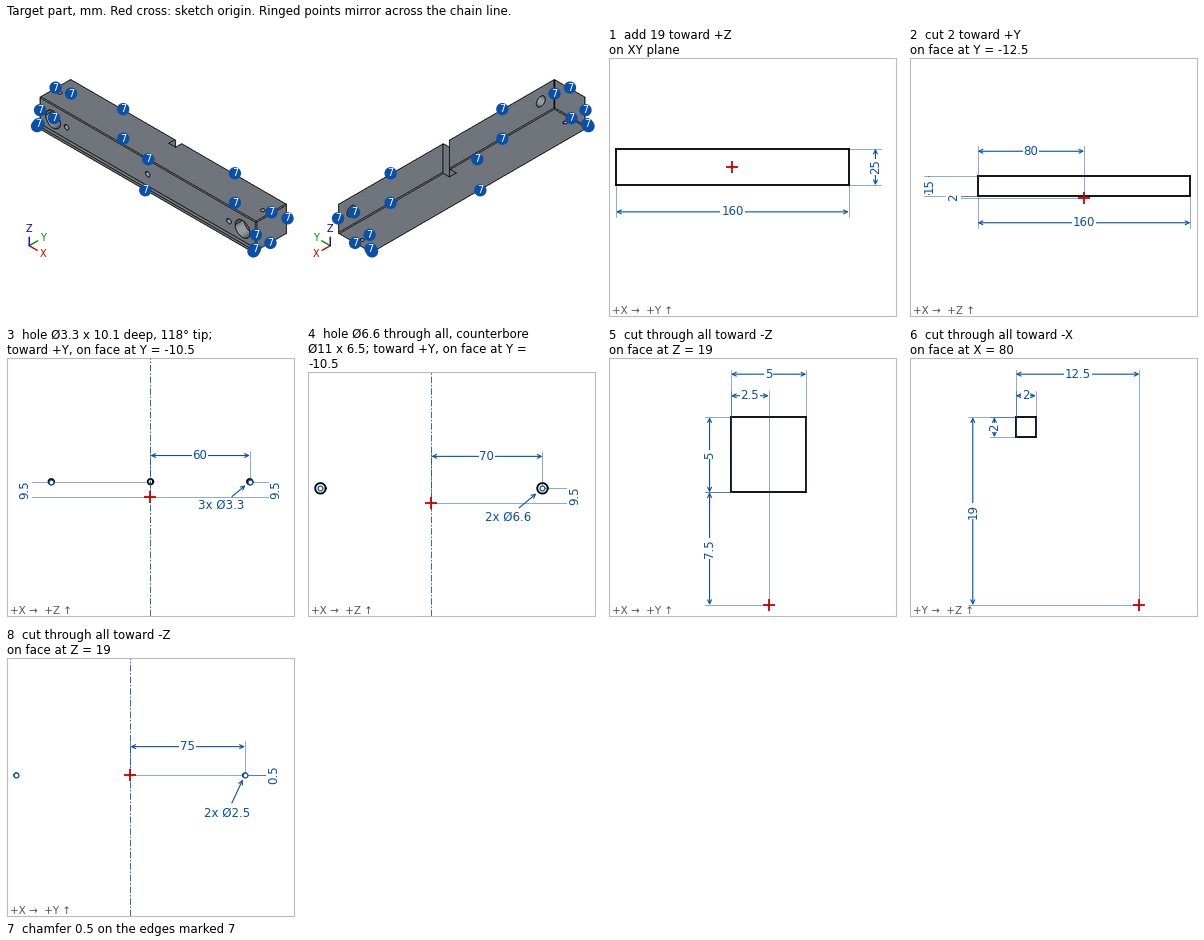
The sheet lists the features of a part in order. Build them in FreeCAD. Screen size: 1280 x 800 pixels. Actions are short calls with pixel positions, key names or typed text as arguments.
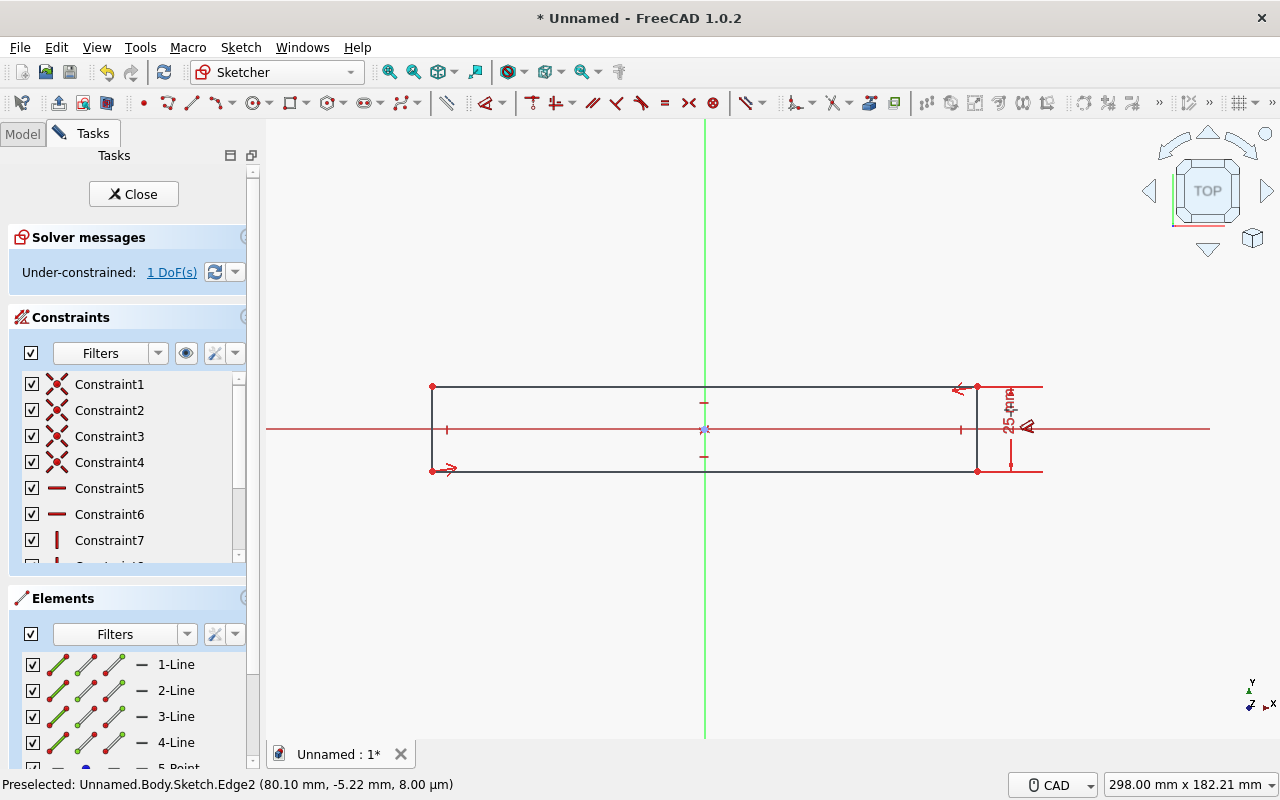
click(596, 472)
click(579, 506)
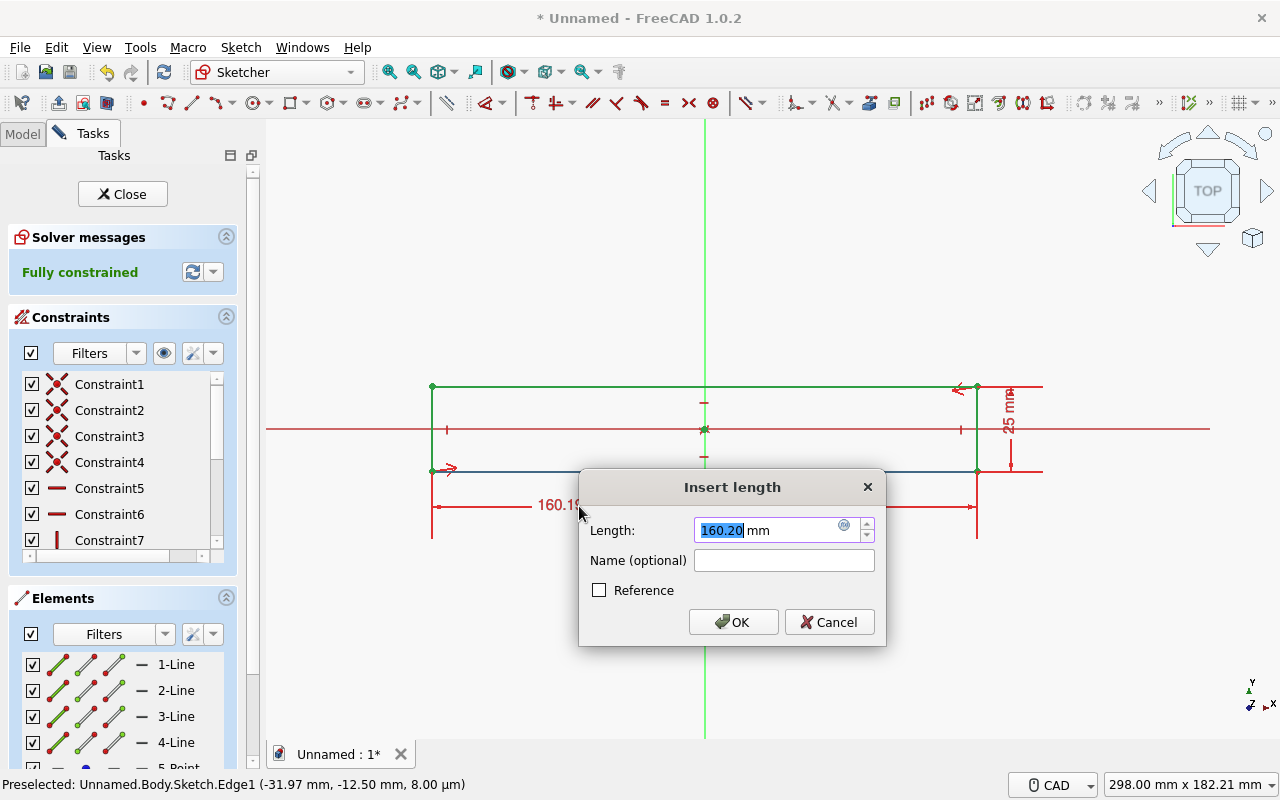
text(160)
key(Return)
key(Escape)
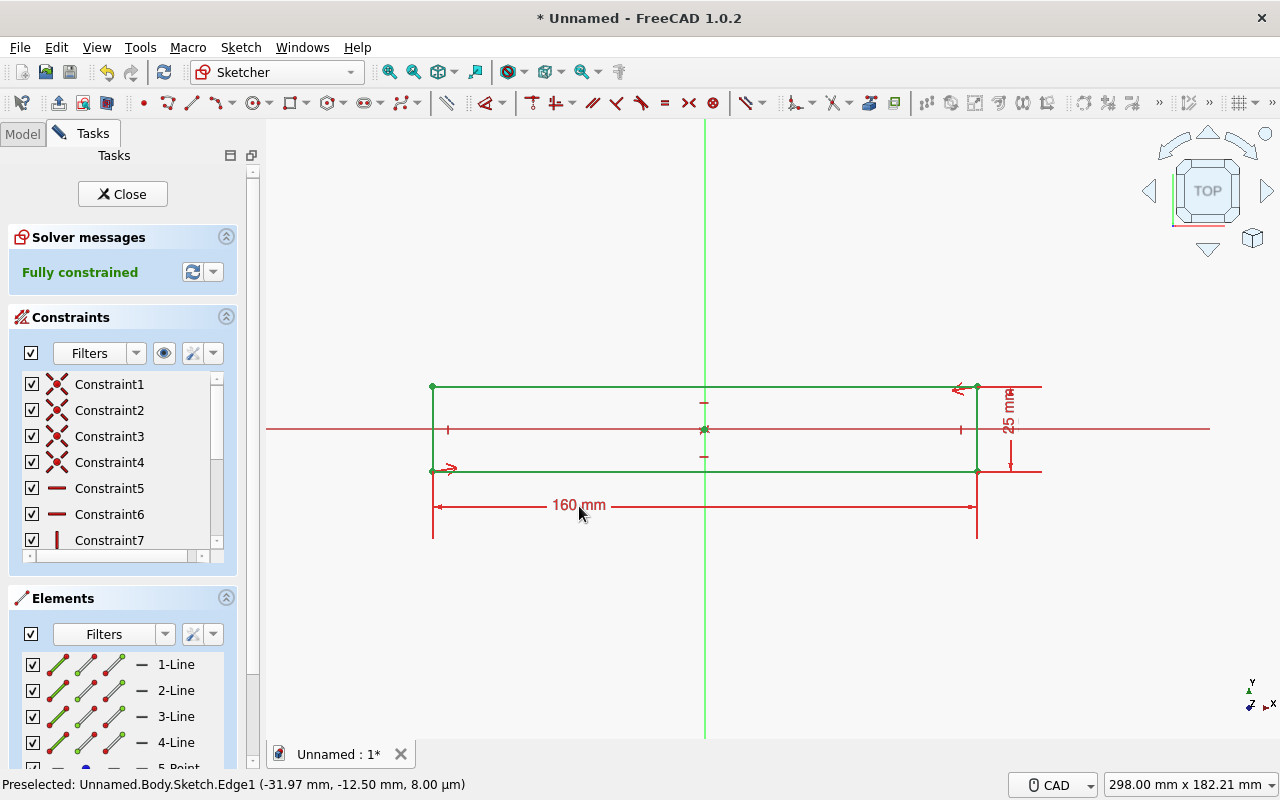
click(123, 194)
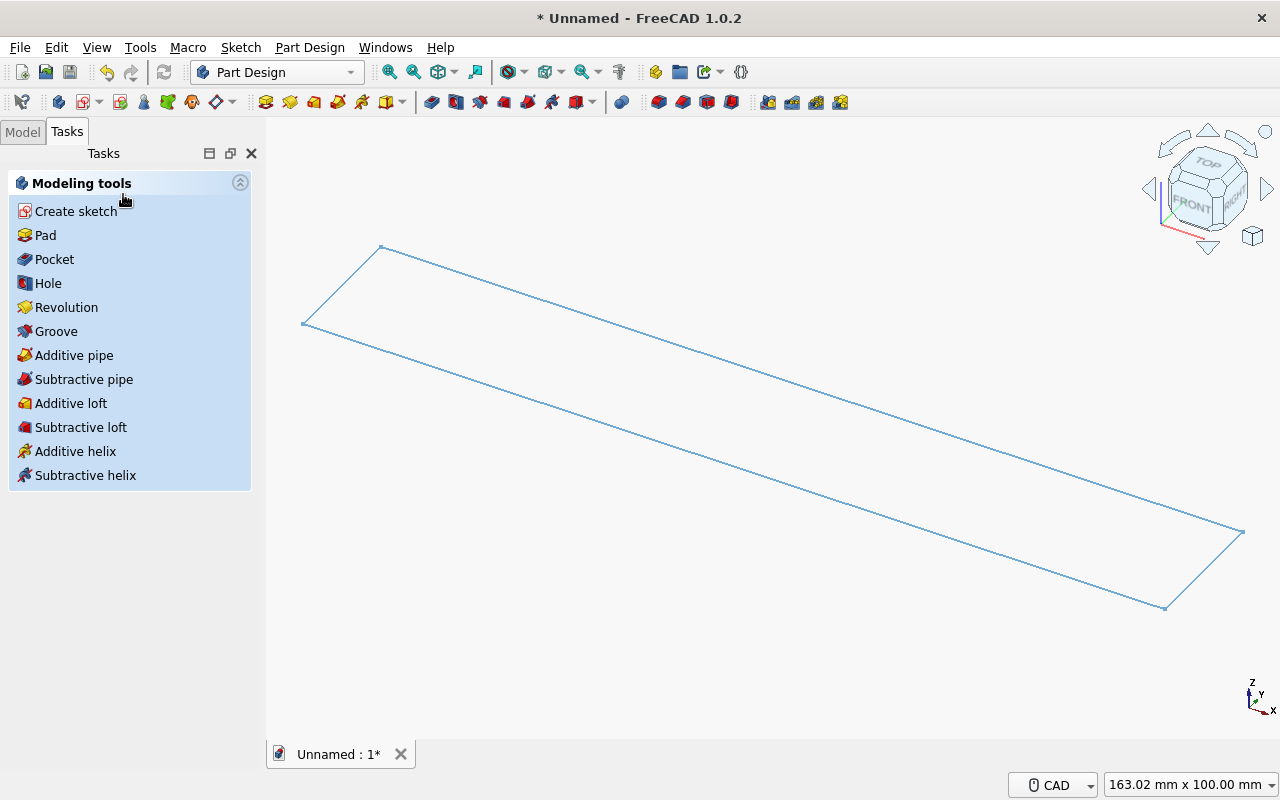
click(266, 102)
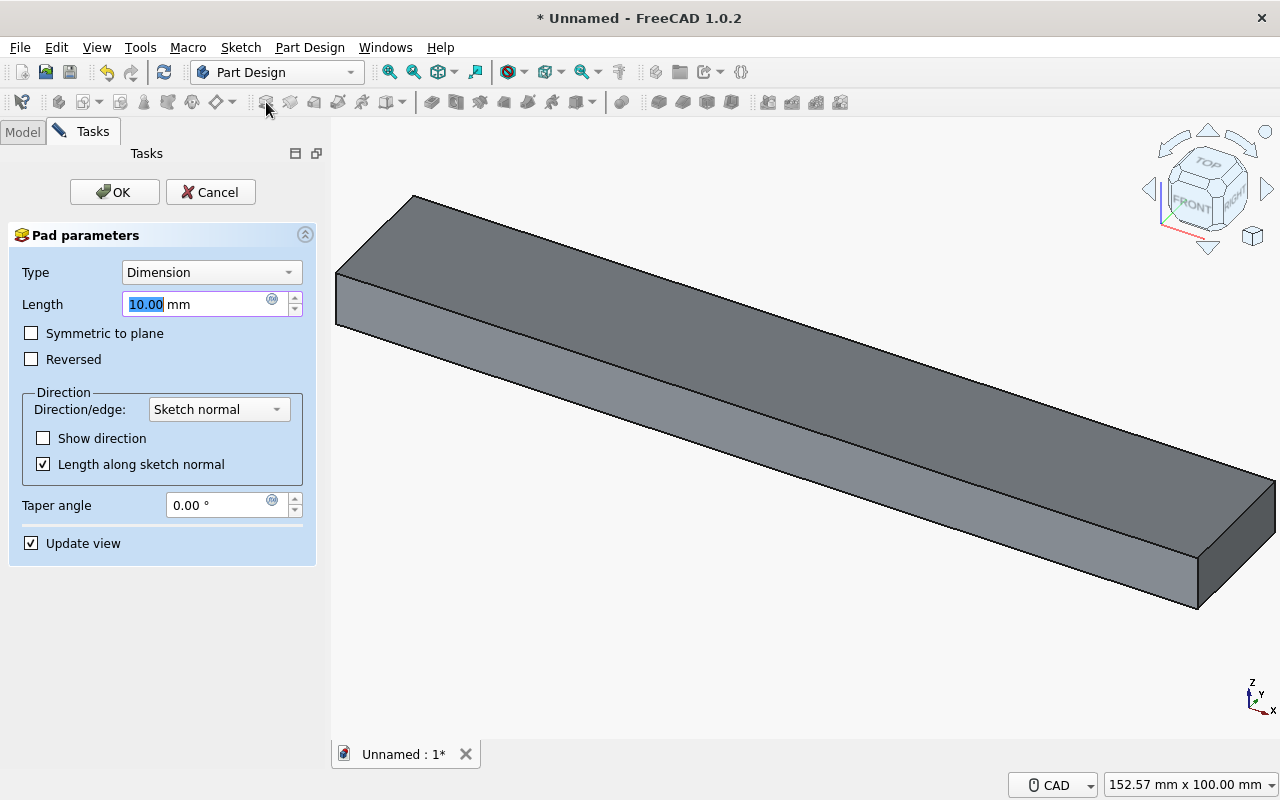
text(19)
key(Tab)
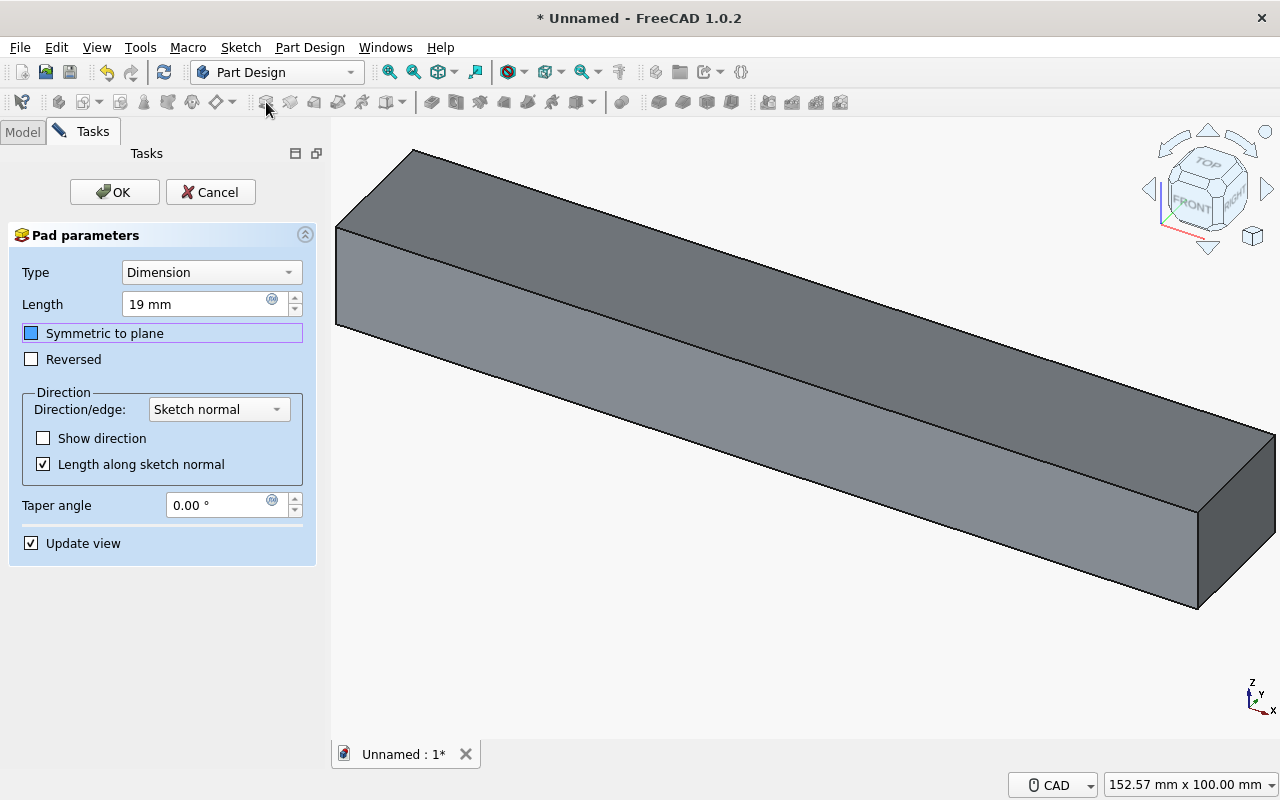
click(115, 192)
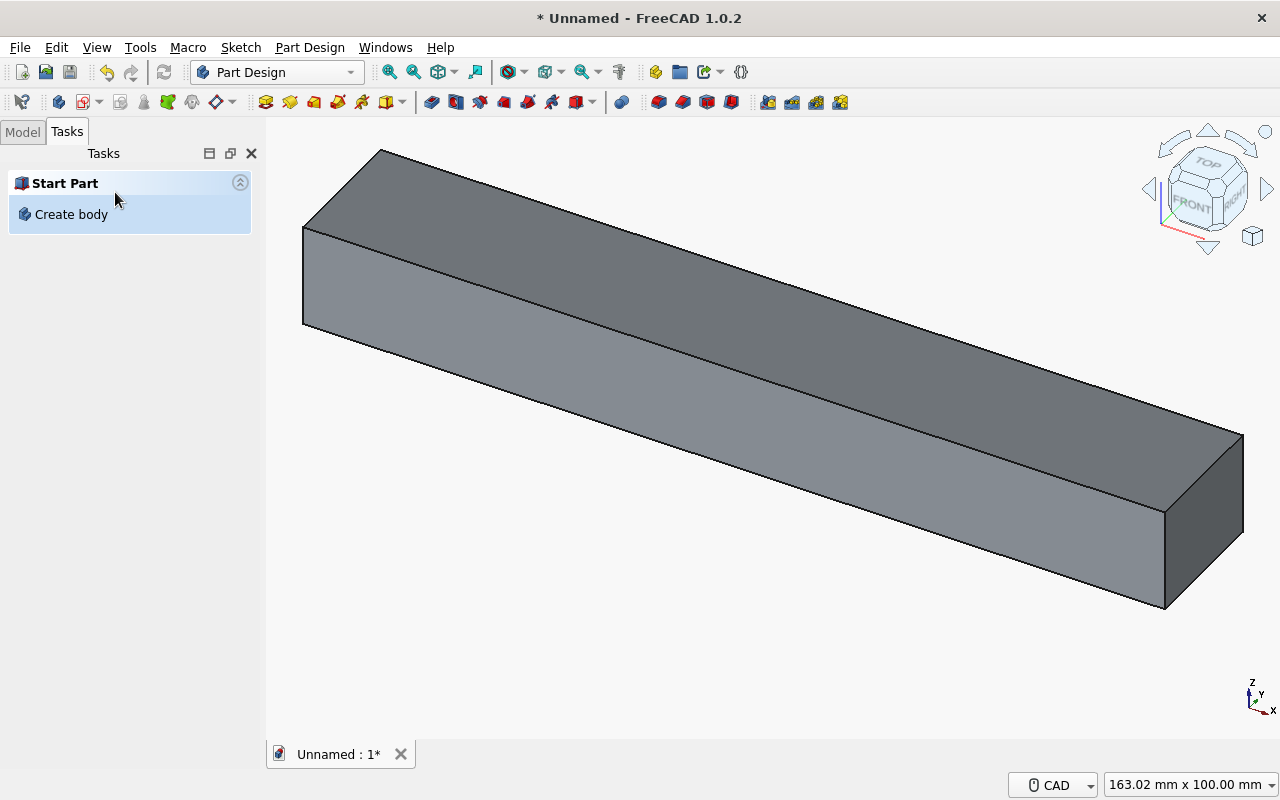
click(1103, 540)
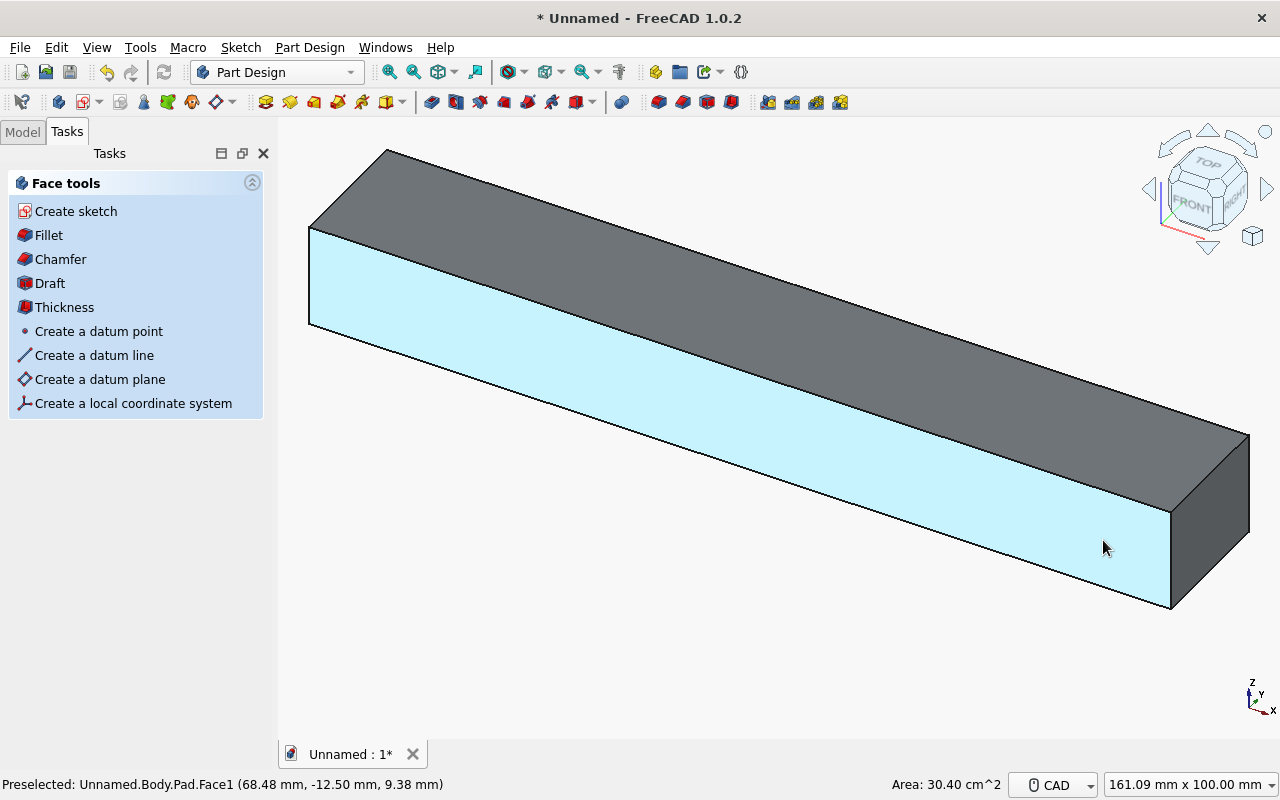
click(84, 102)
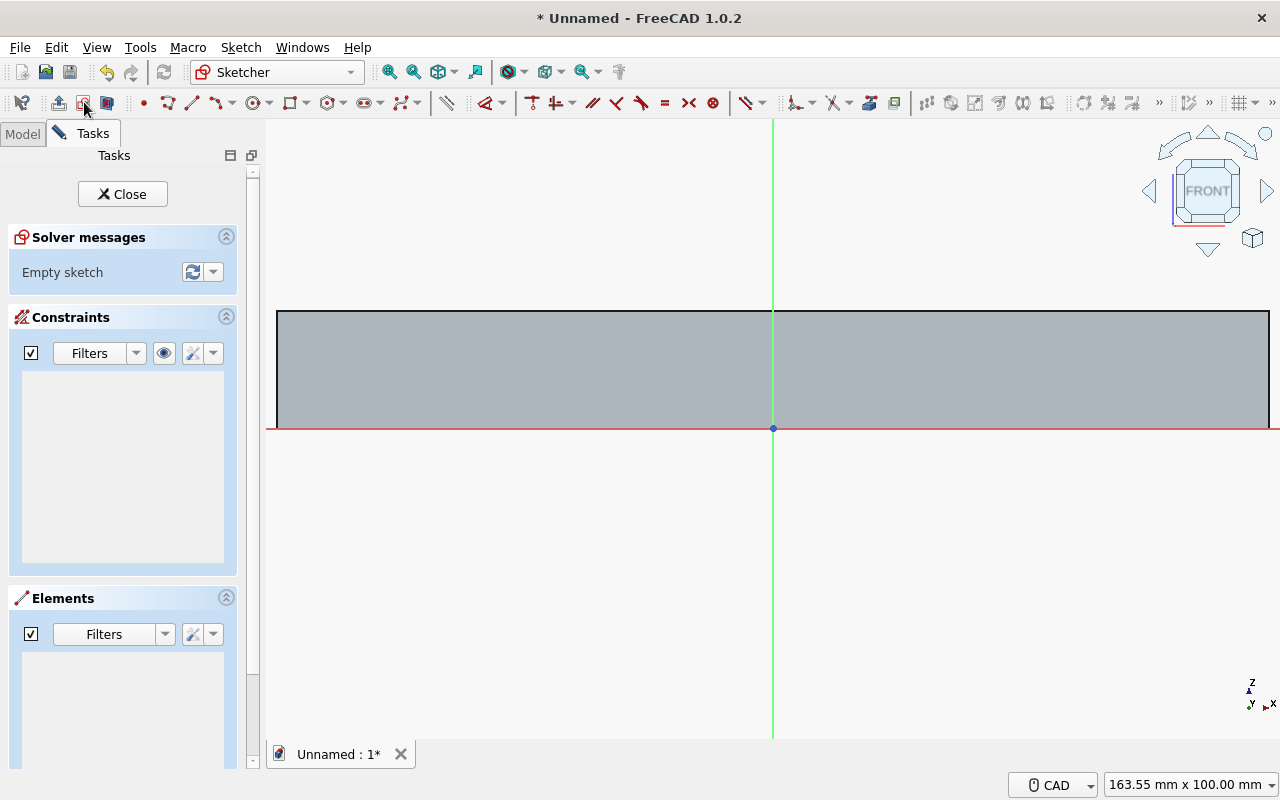
scroll(621, 493, down, 3)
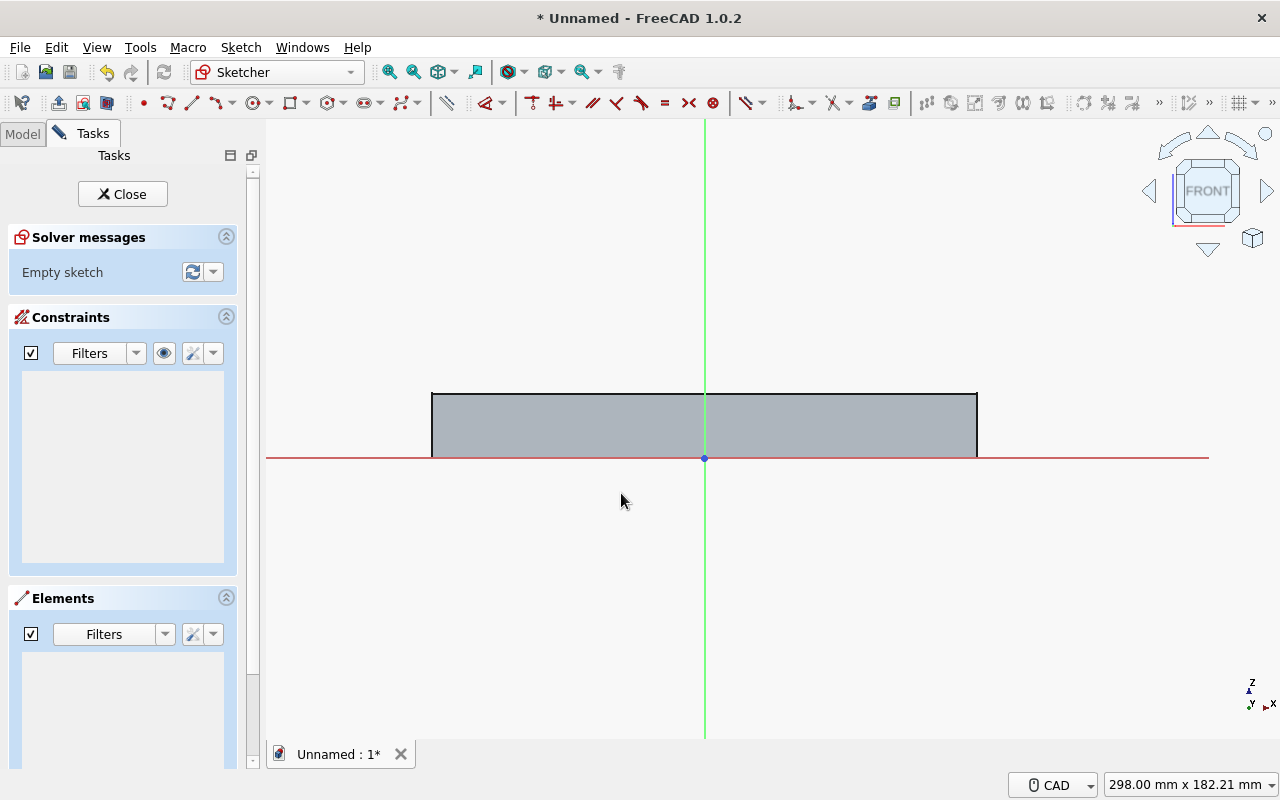
click(290, 104)